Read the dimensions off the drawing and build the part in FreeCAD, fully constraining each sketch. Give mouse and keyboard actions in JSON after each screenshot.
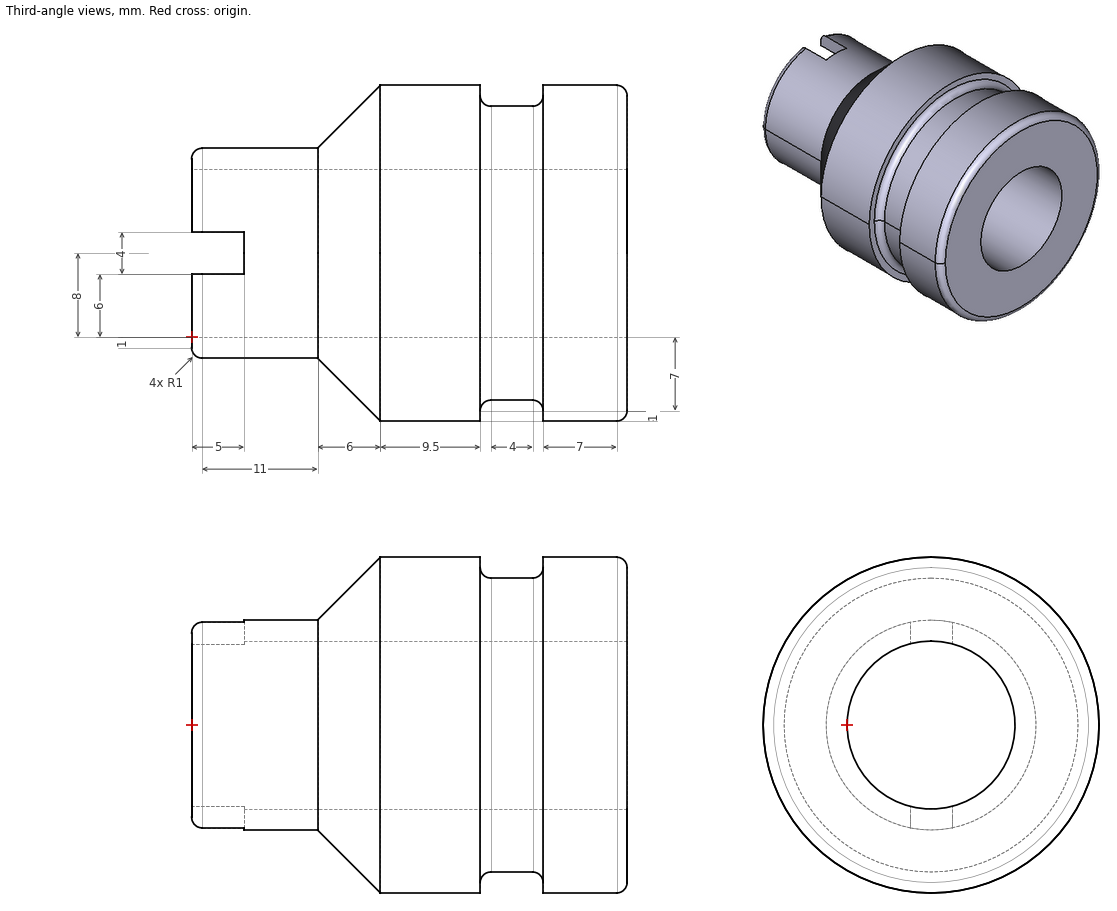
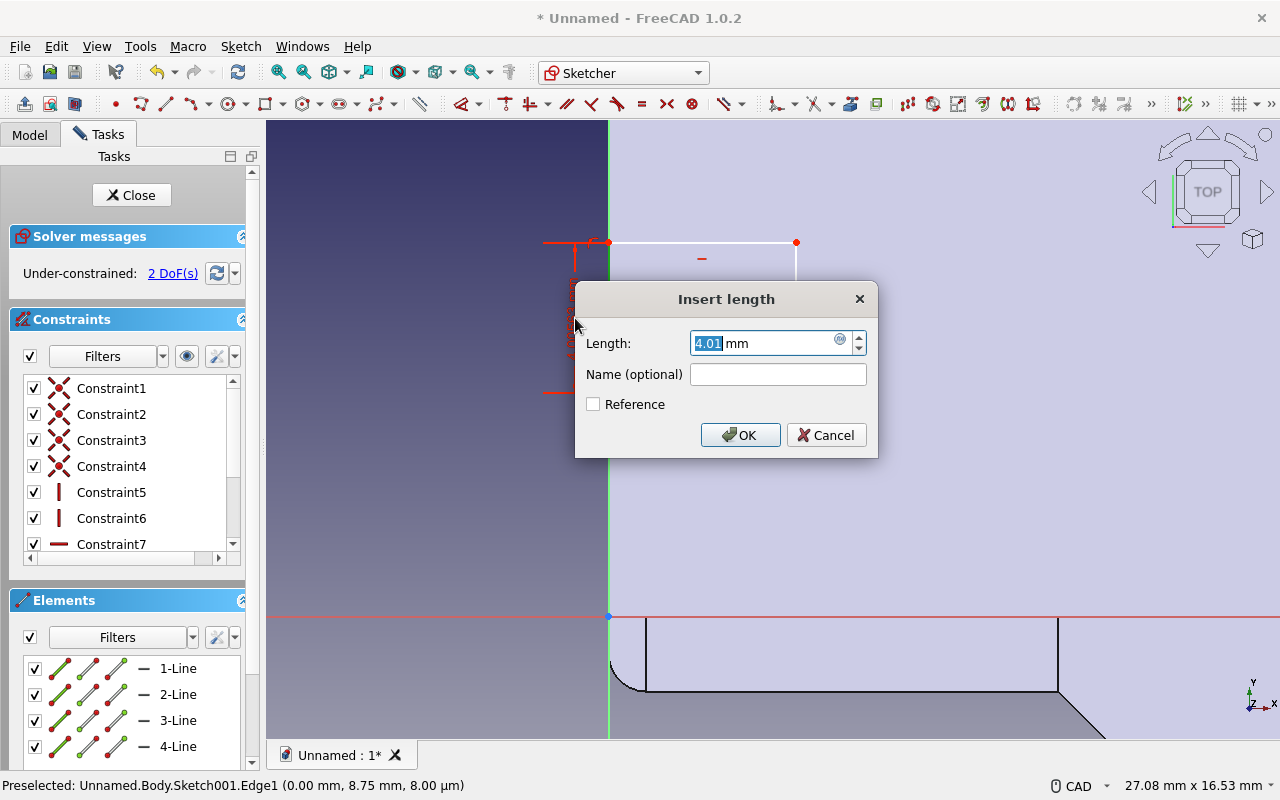
{"action": "type", "text": "4"}
{"action": "key", "text": "Return"}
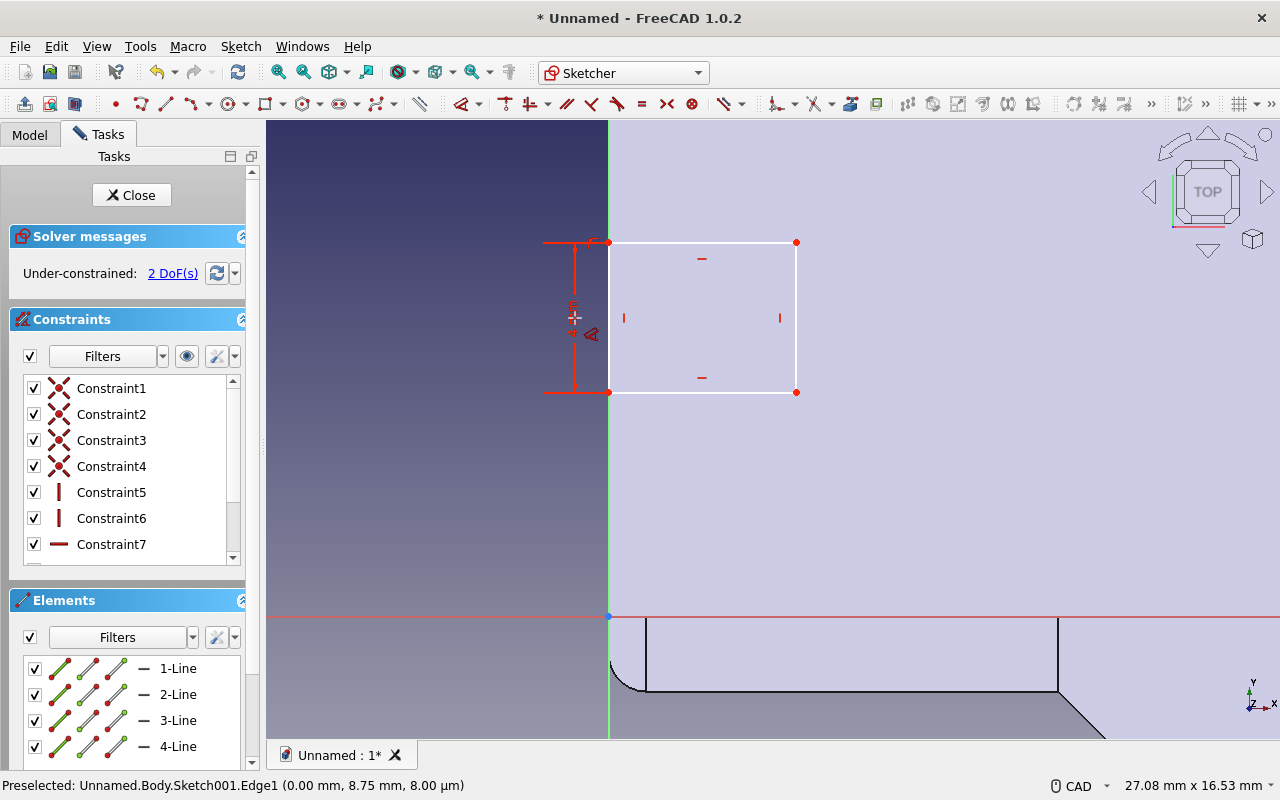
{"action": "left_click", "coordinate": [665, 393]}
{"action": "left_click", "coordinate": [702, 359]}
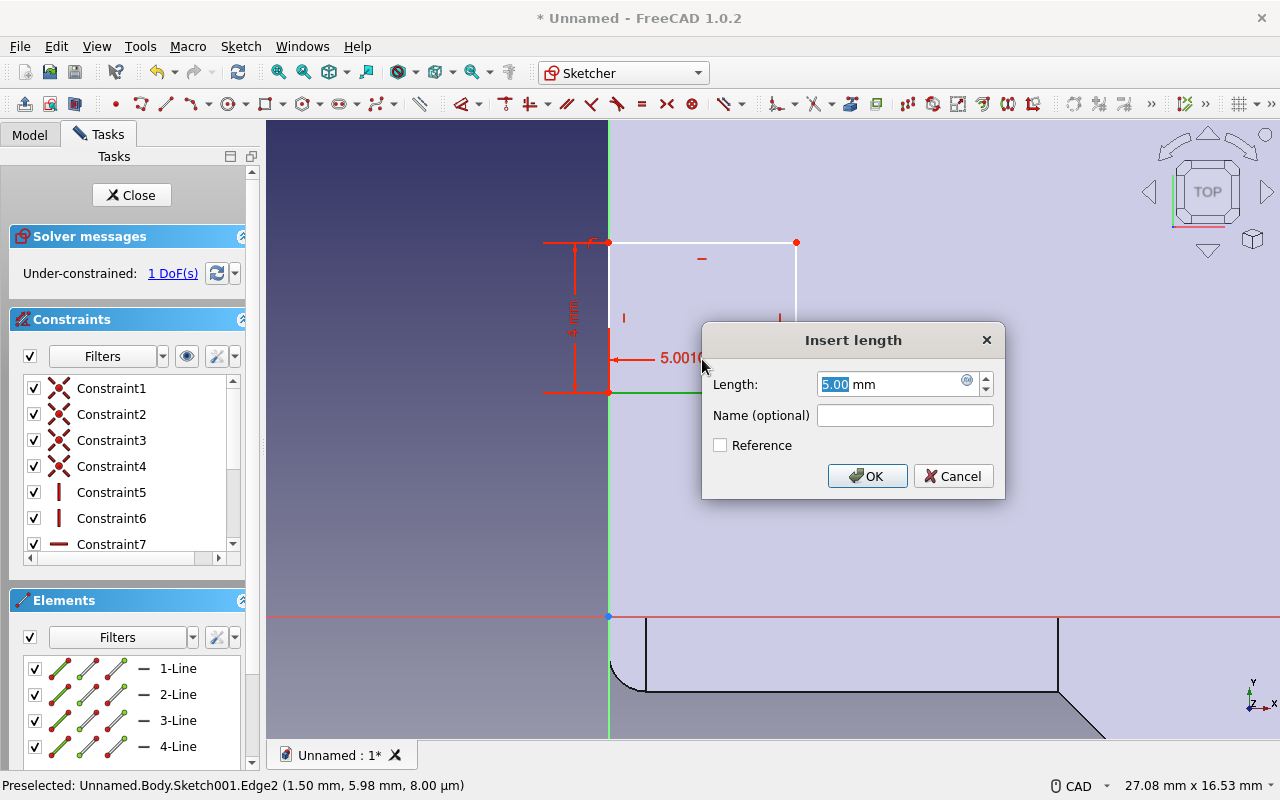
{"action": "type", "text": "5"}
{"action": "key", "text": "Return"}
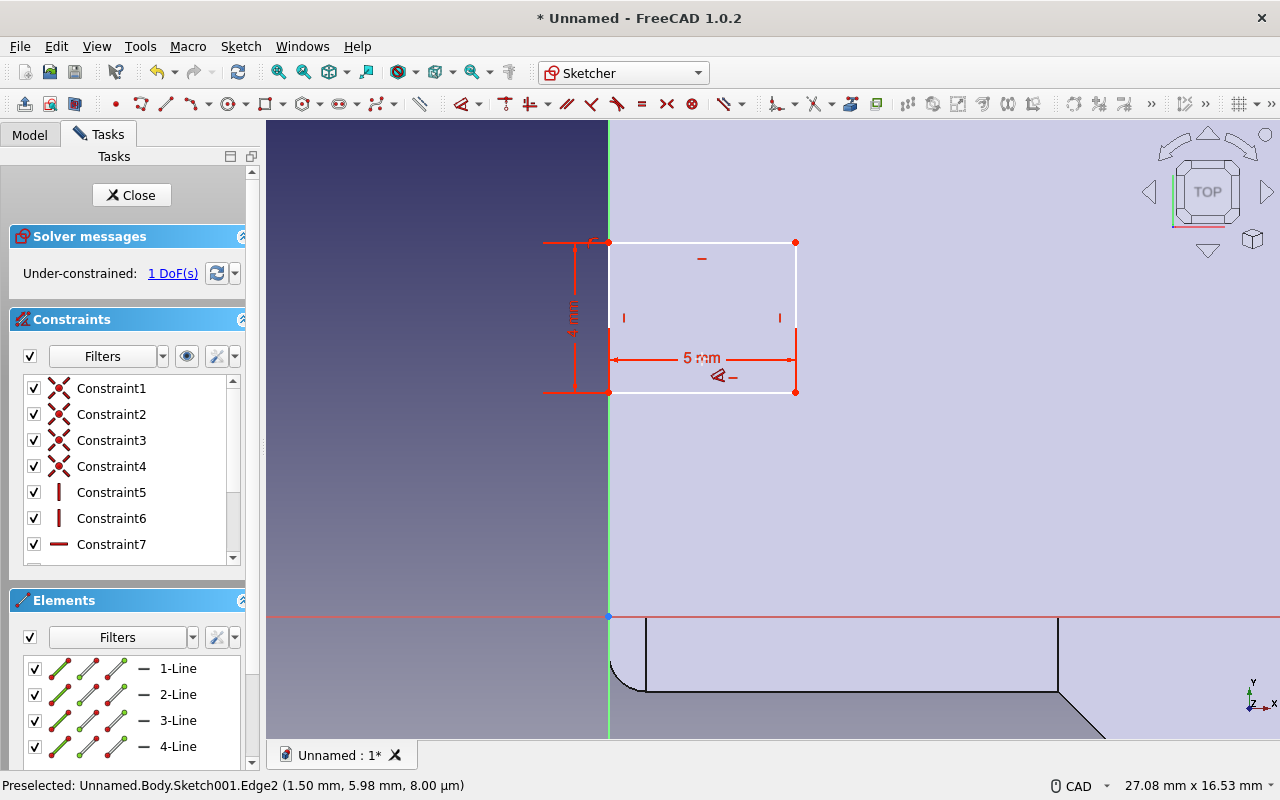
{"action": "left_click", "coordinate": [609, 393]}
{"action": "left_click", "coordinate": [575, 505]}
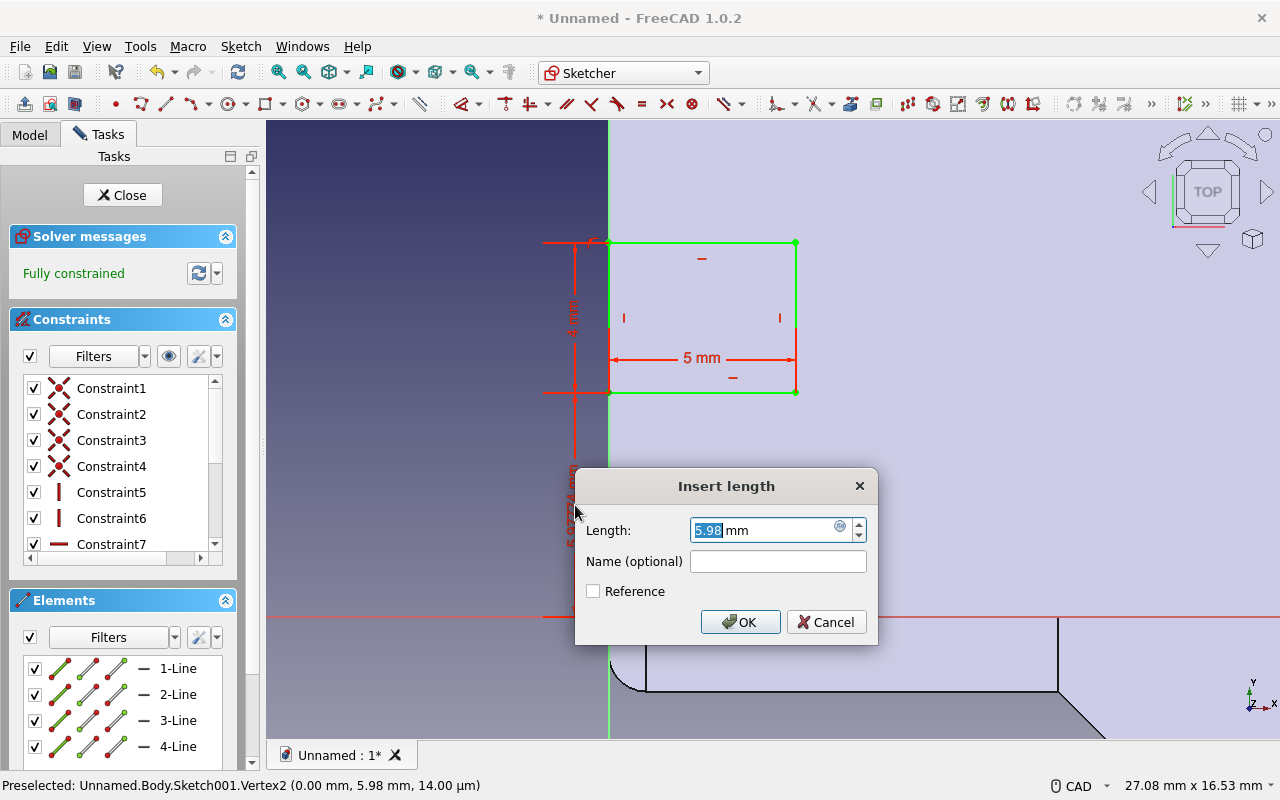
{"action": "type", "text": "6"}
{"action": "key", "text": "Return"}
{"action": "key", "text": "Escape"}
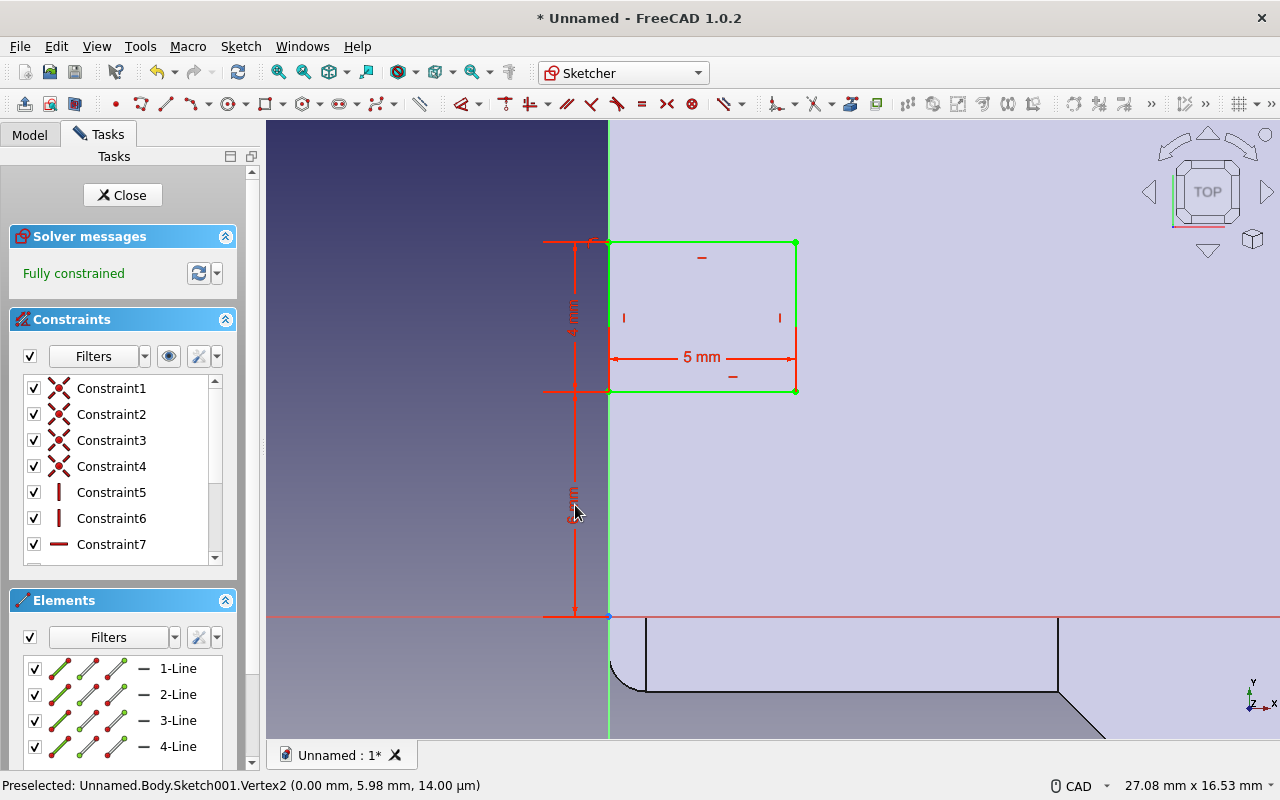
{"action": "left_click", "coordinate": [123, 195]}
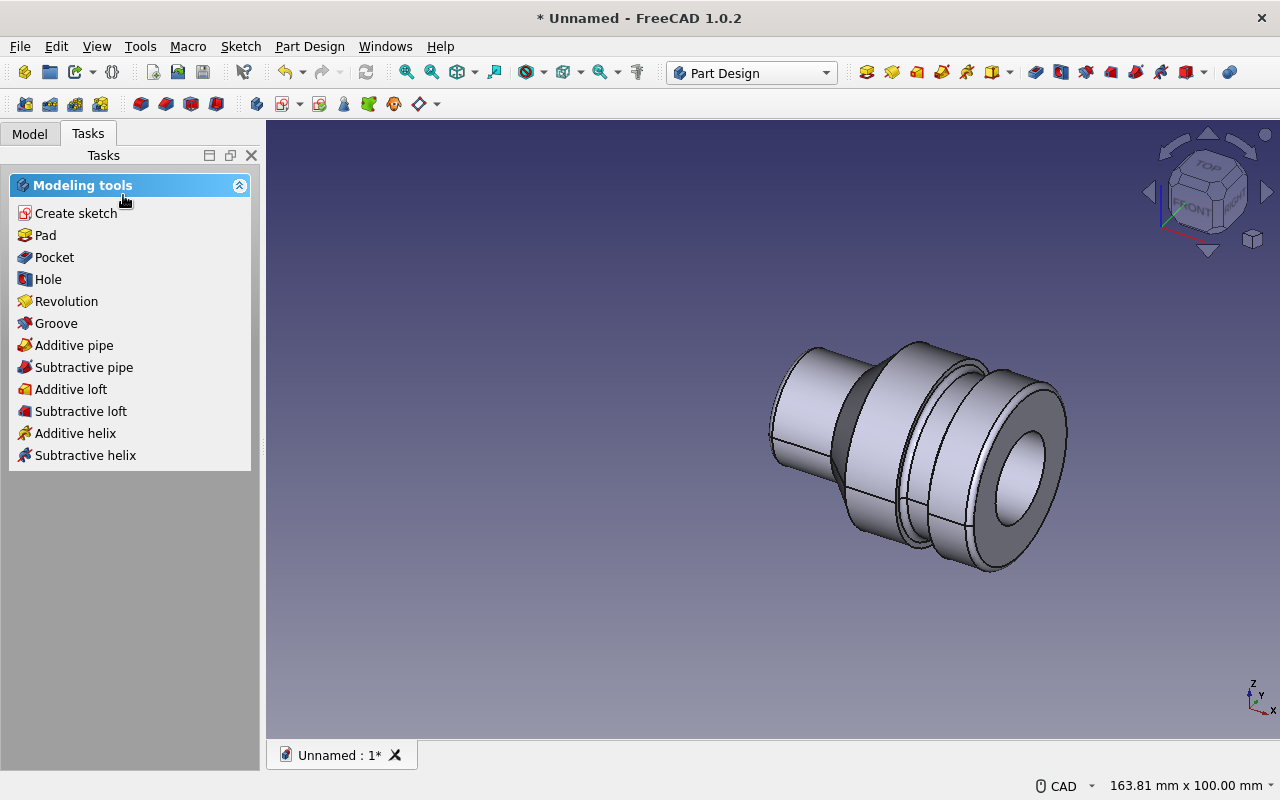
{"action": "left_click", "coordinate": [1036, 72]}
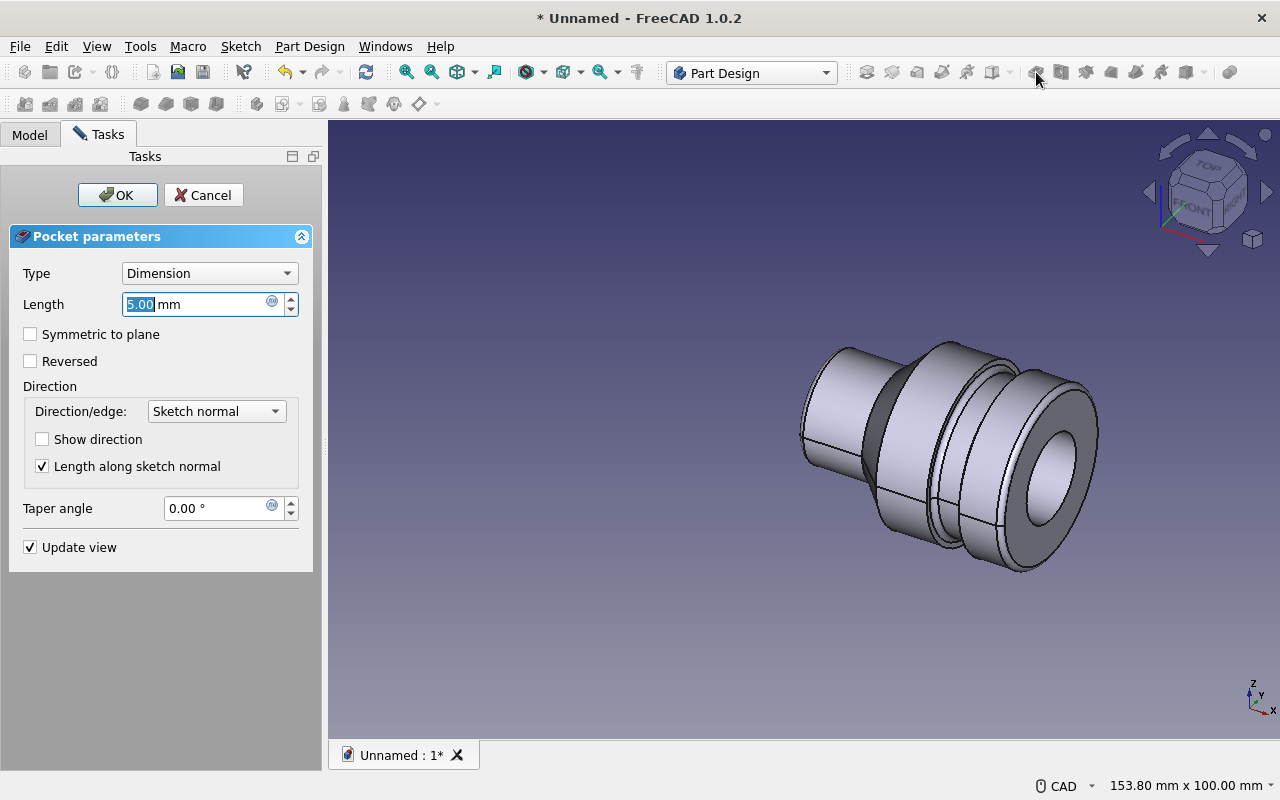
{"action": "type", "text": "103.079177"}
{"action": "key", "text": "Tab"}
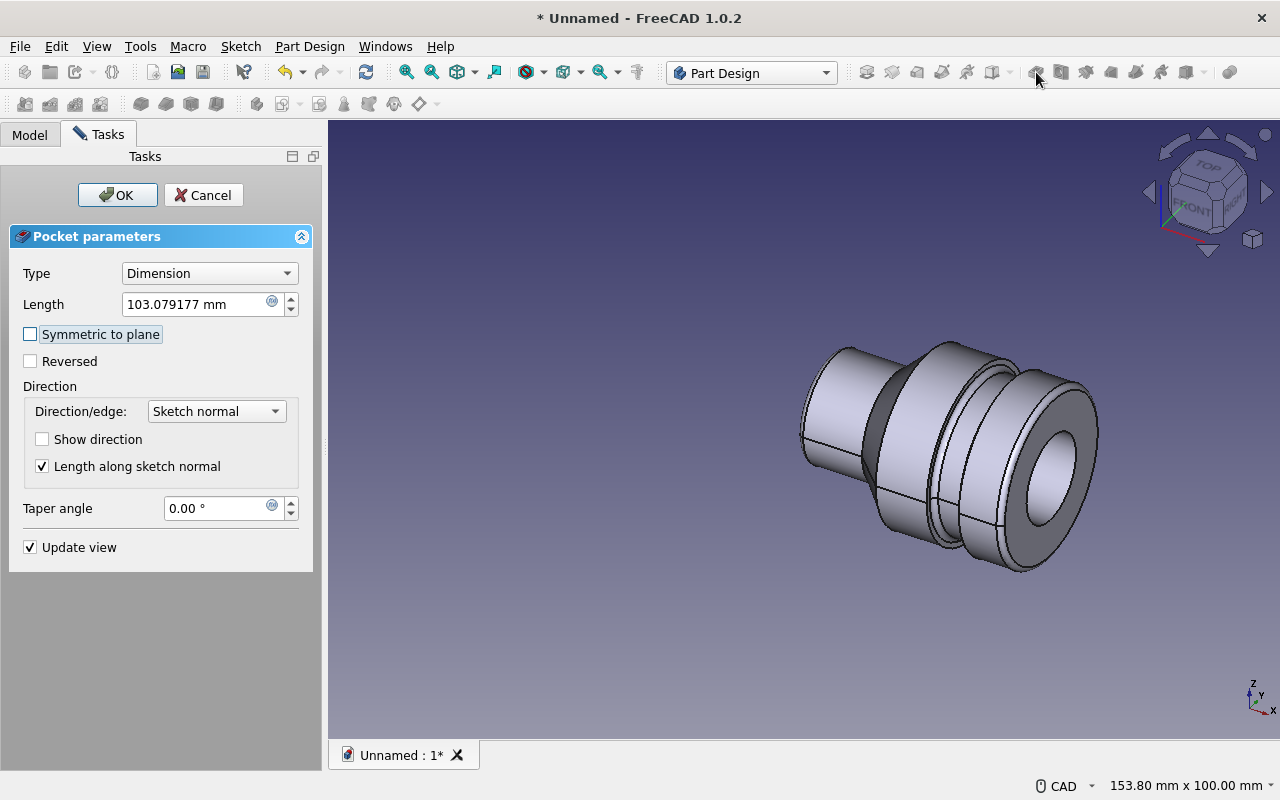
{"action": "left_click", "coordinate": [31, 334]}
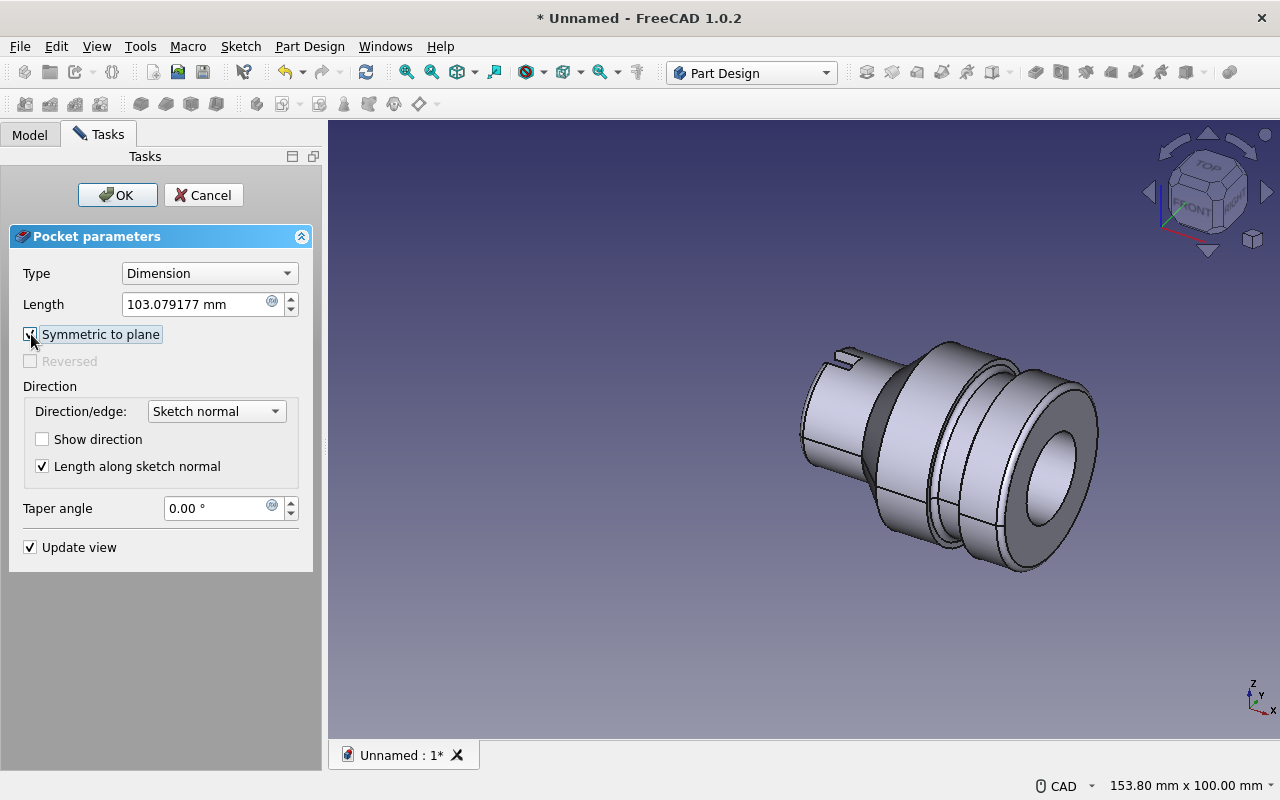
{"action": "left_click", "coordinate": [118, 195]}